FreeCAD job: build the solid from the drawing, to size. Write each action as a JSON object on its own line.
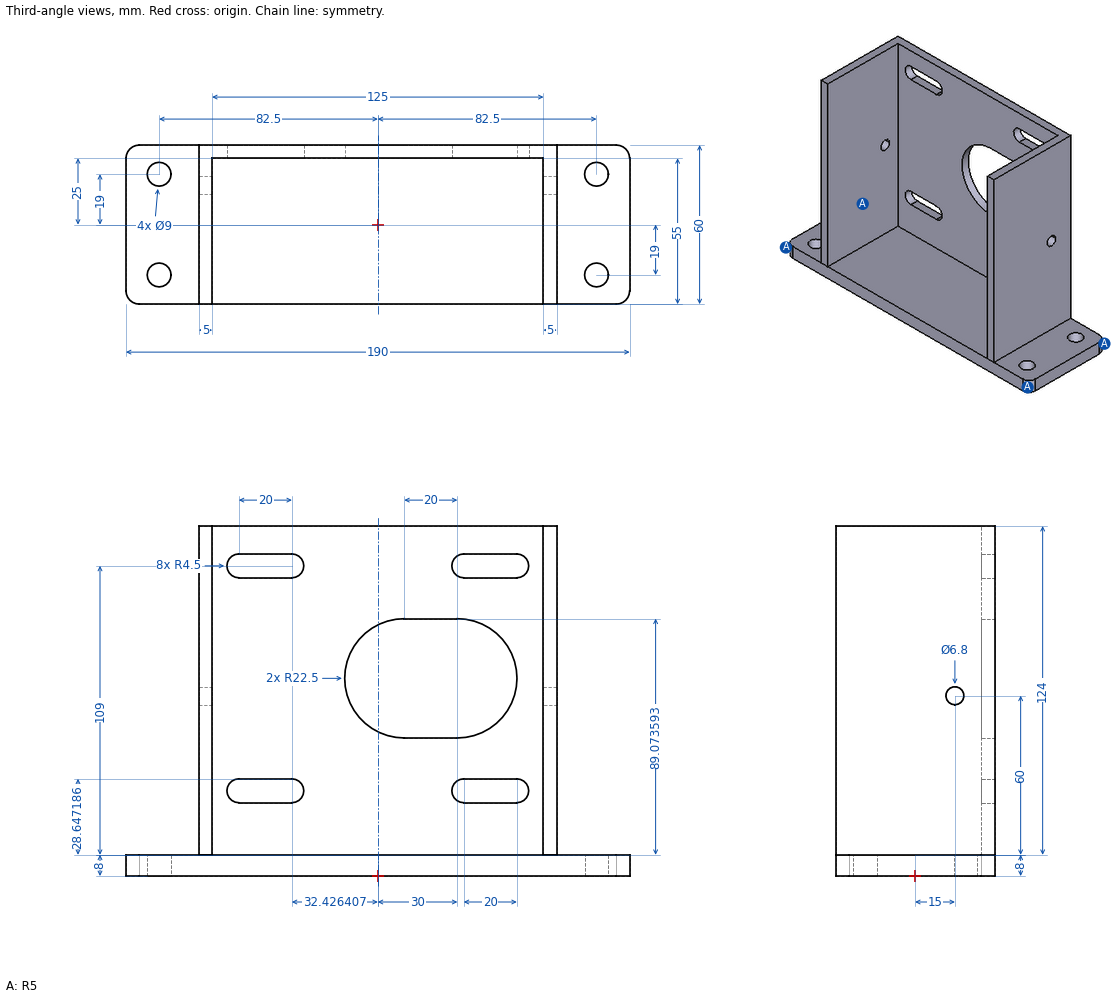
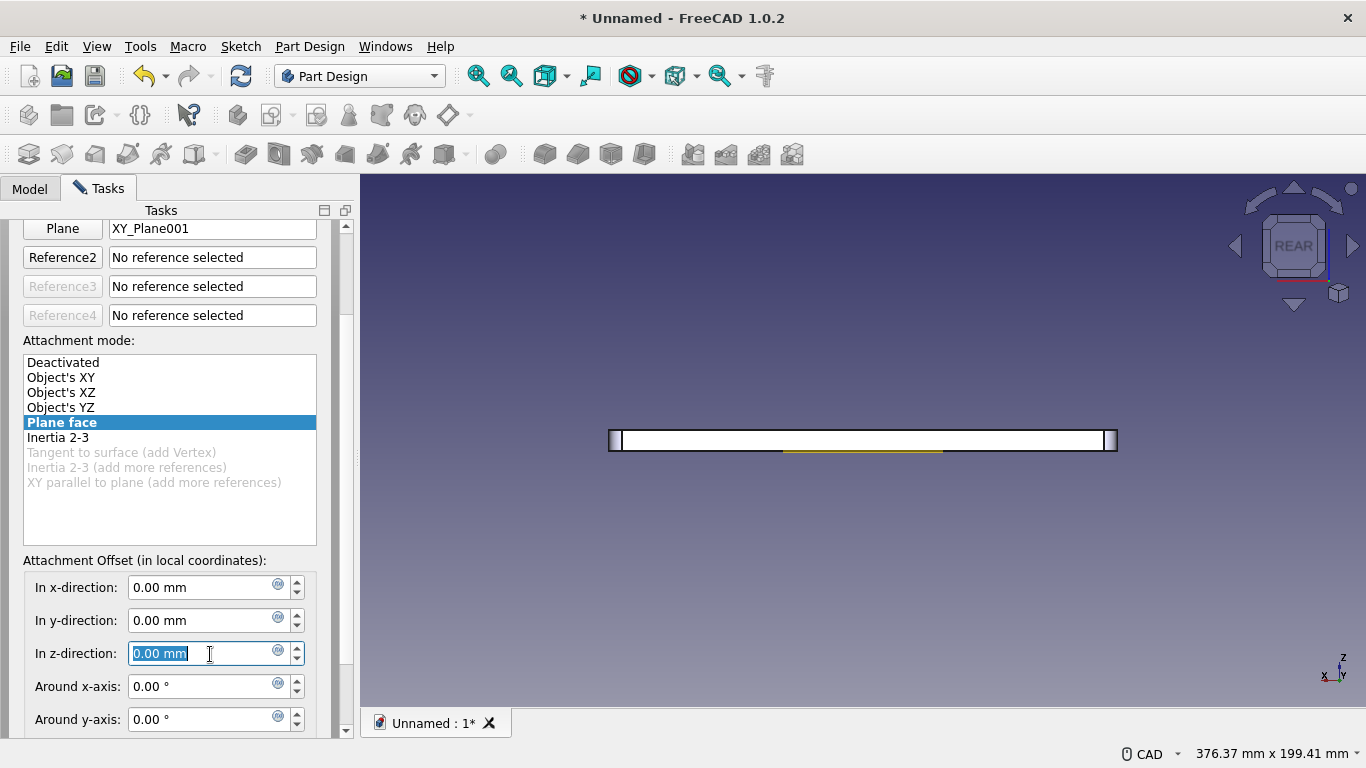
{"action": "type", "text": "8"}
{"action": "key", "text": "Tab"}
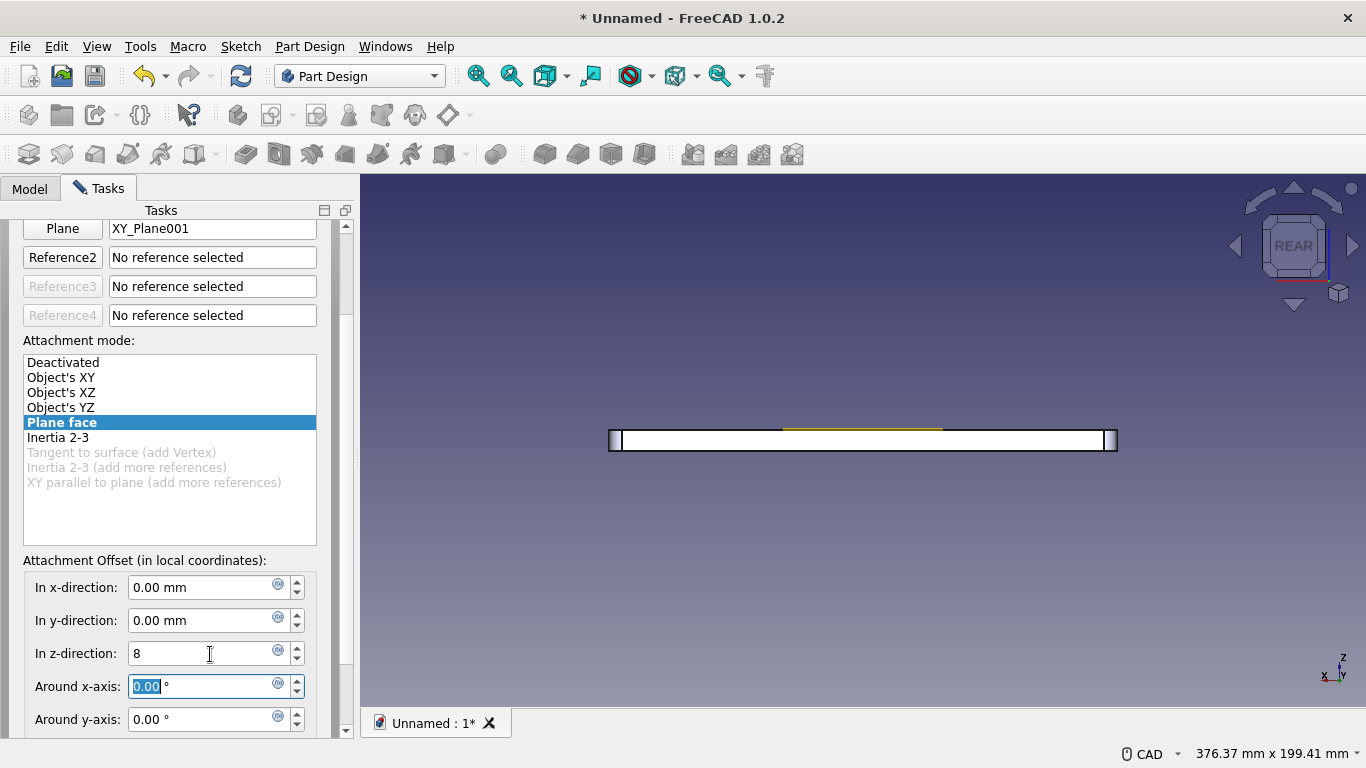
{"action": "scroll", "coordinate": [346, 479], "scroll_direction": "up", "scroll_amount": 3}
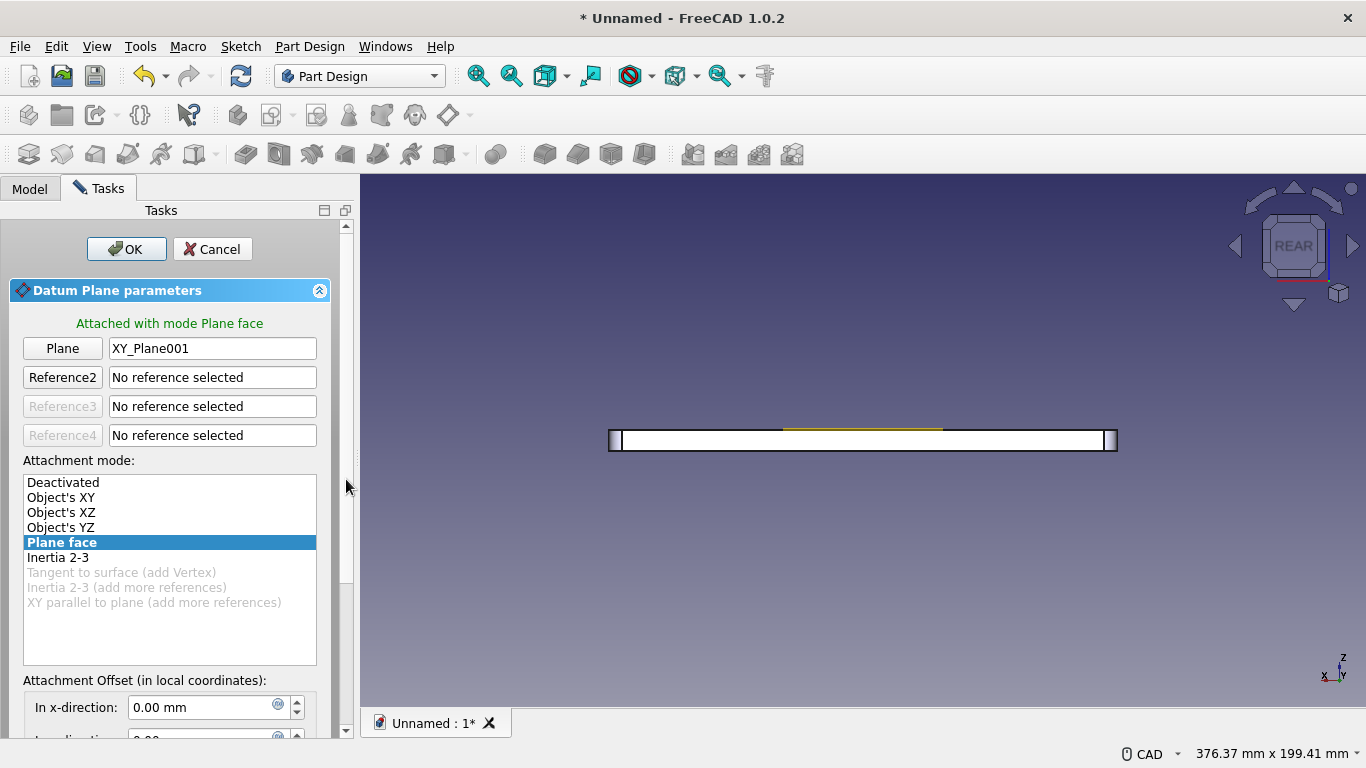
{"action": "left_click", "coordinate": [127, 249]}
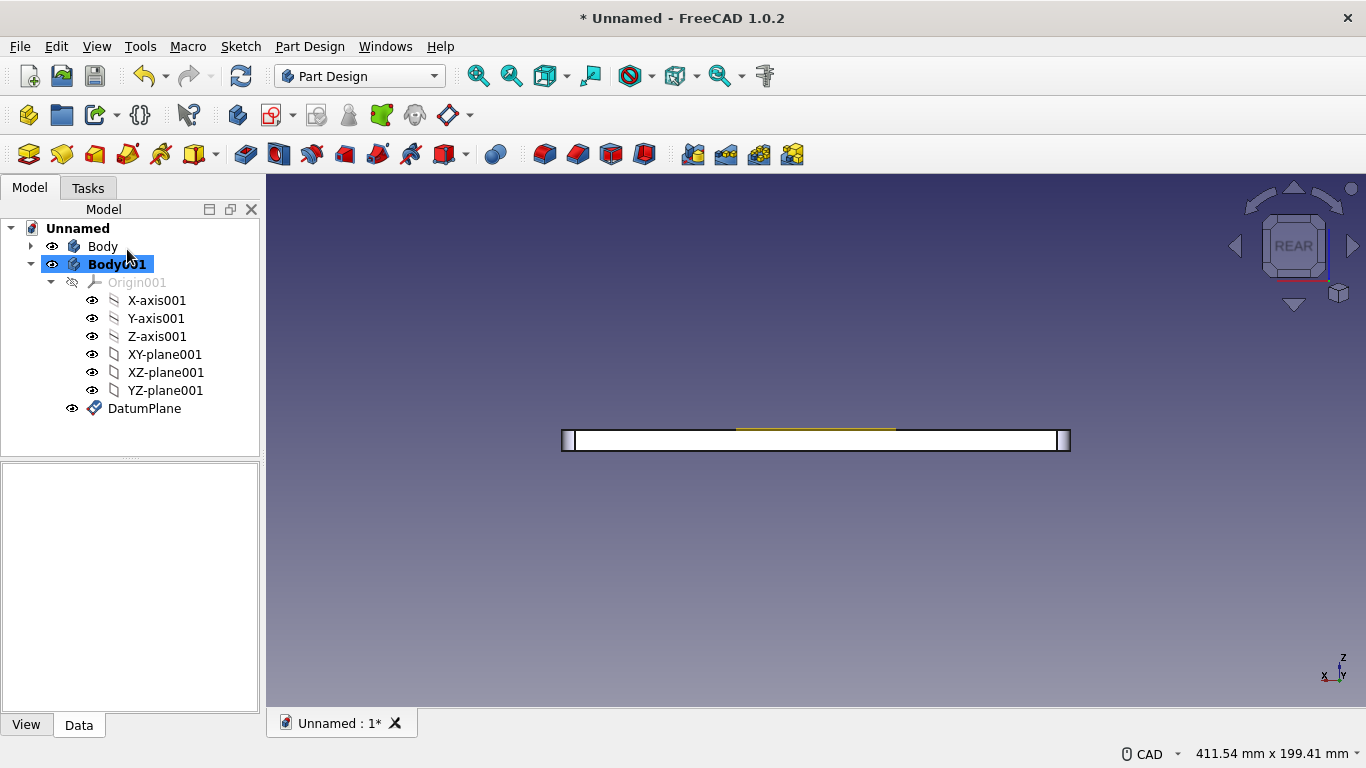
{"action": "left_click", "coordinate": [117, 408]}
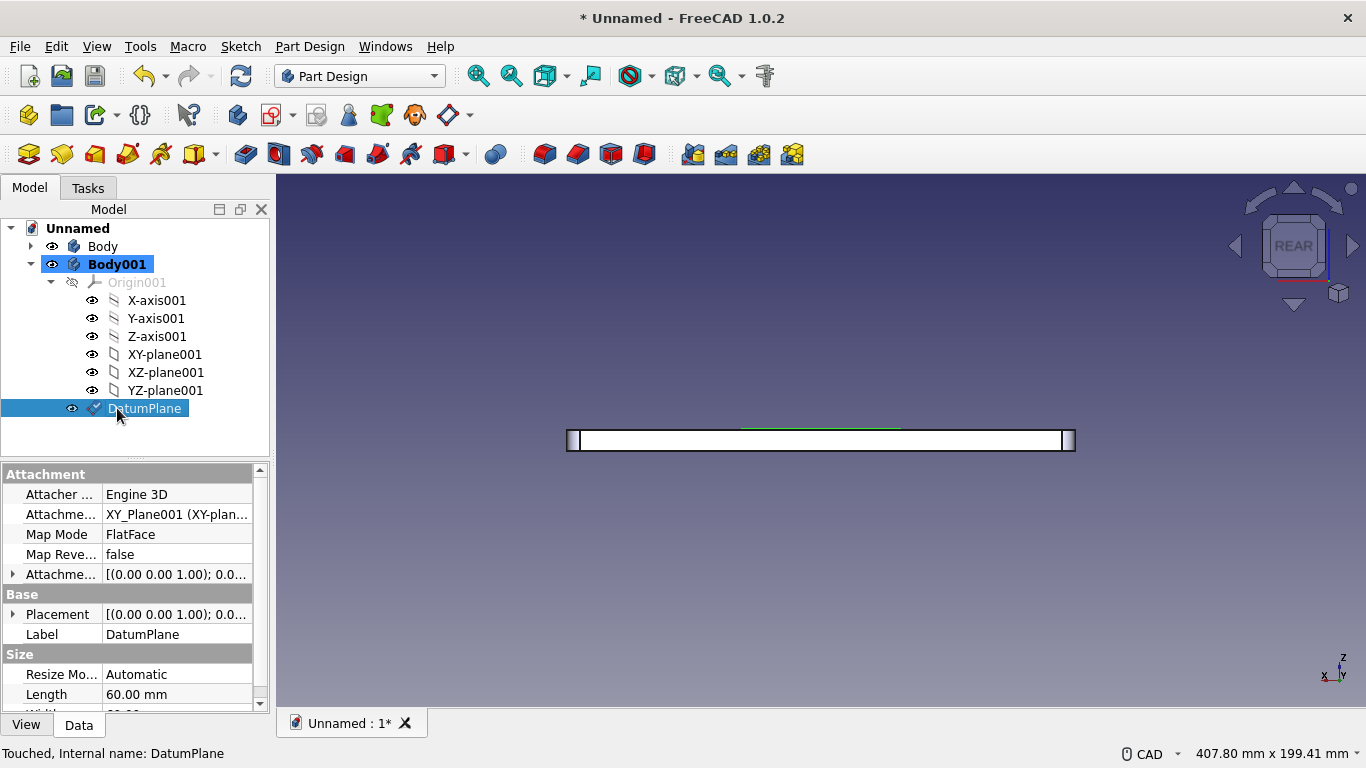
{"action": "left_click", "coordinate": [270, 116]}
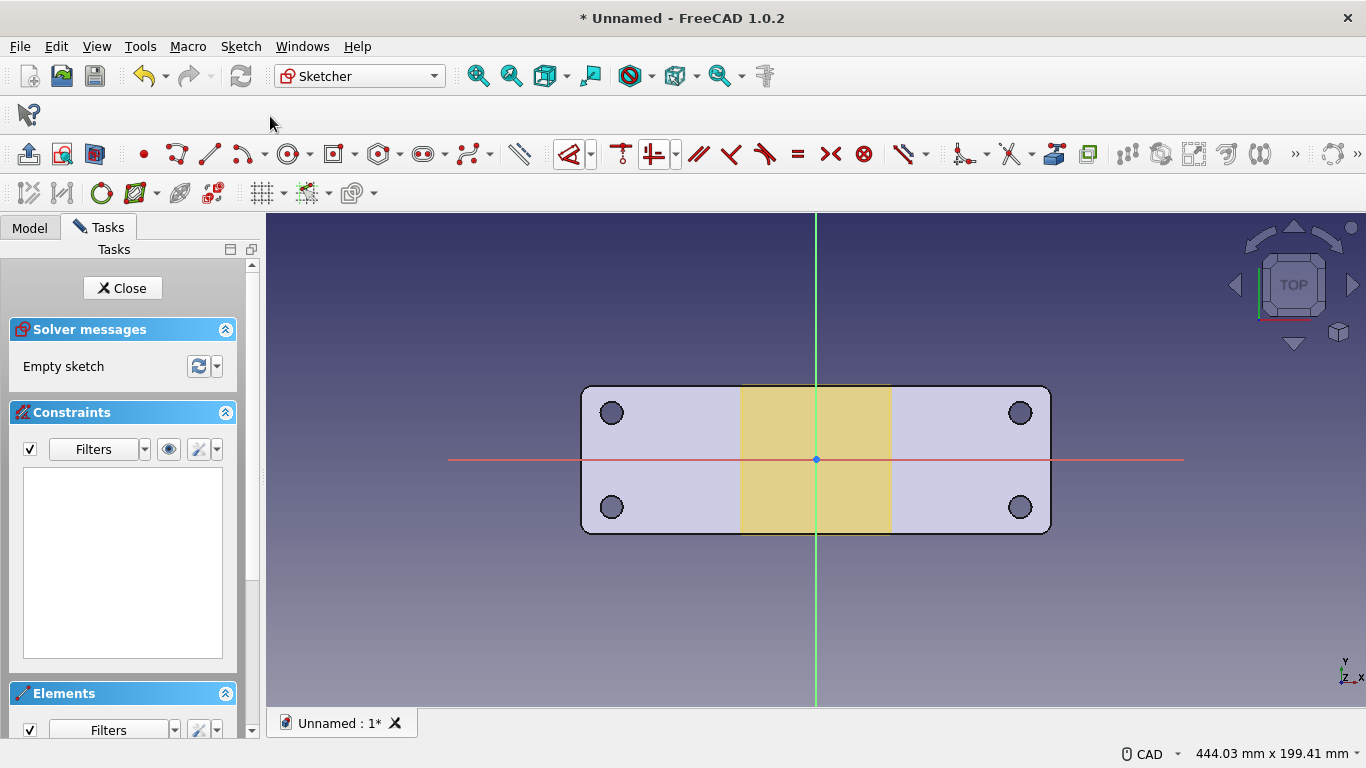
{"action": "scroll", "coordinate": [899, 460], "scroll_direction": "up", "scroll_amount": 3}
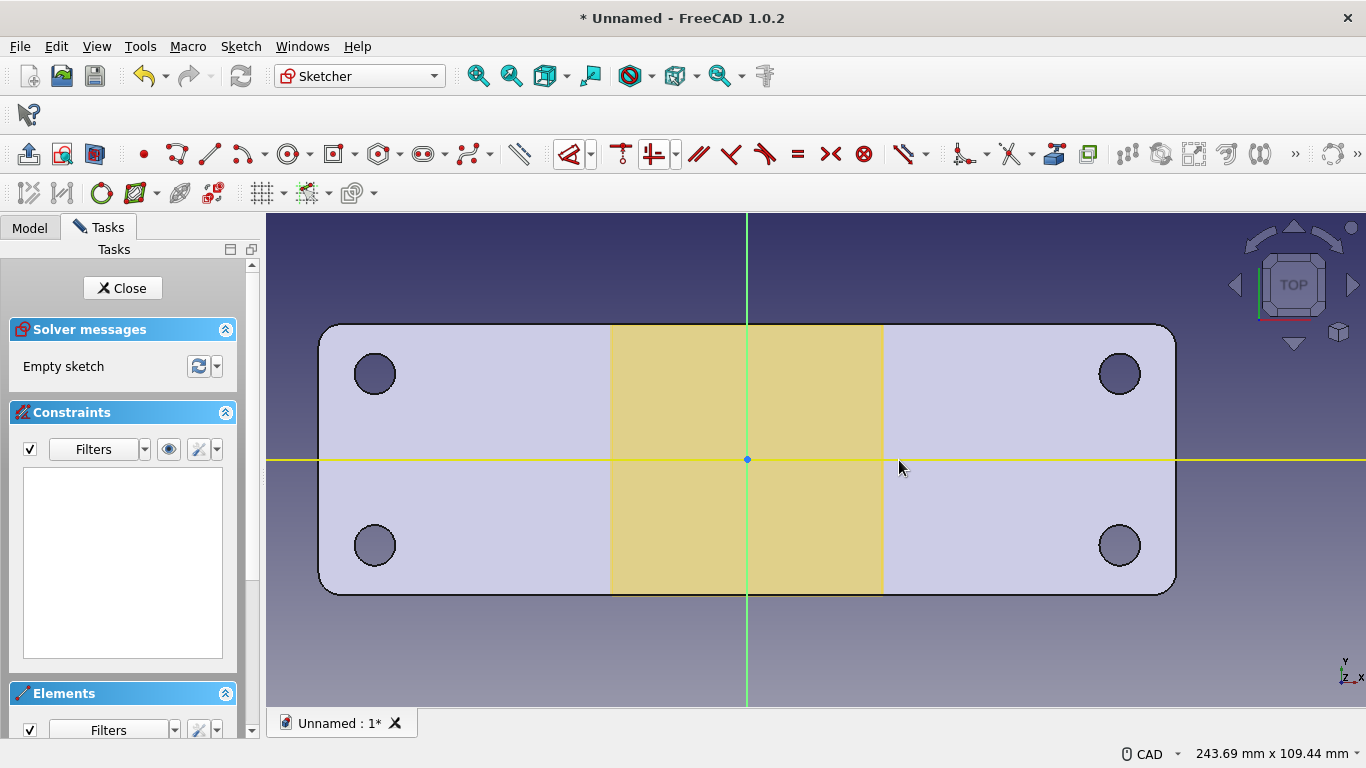
{"action": "left_click", "coordinate": [177, 154]}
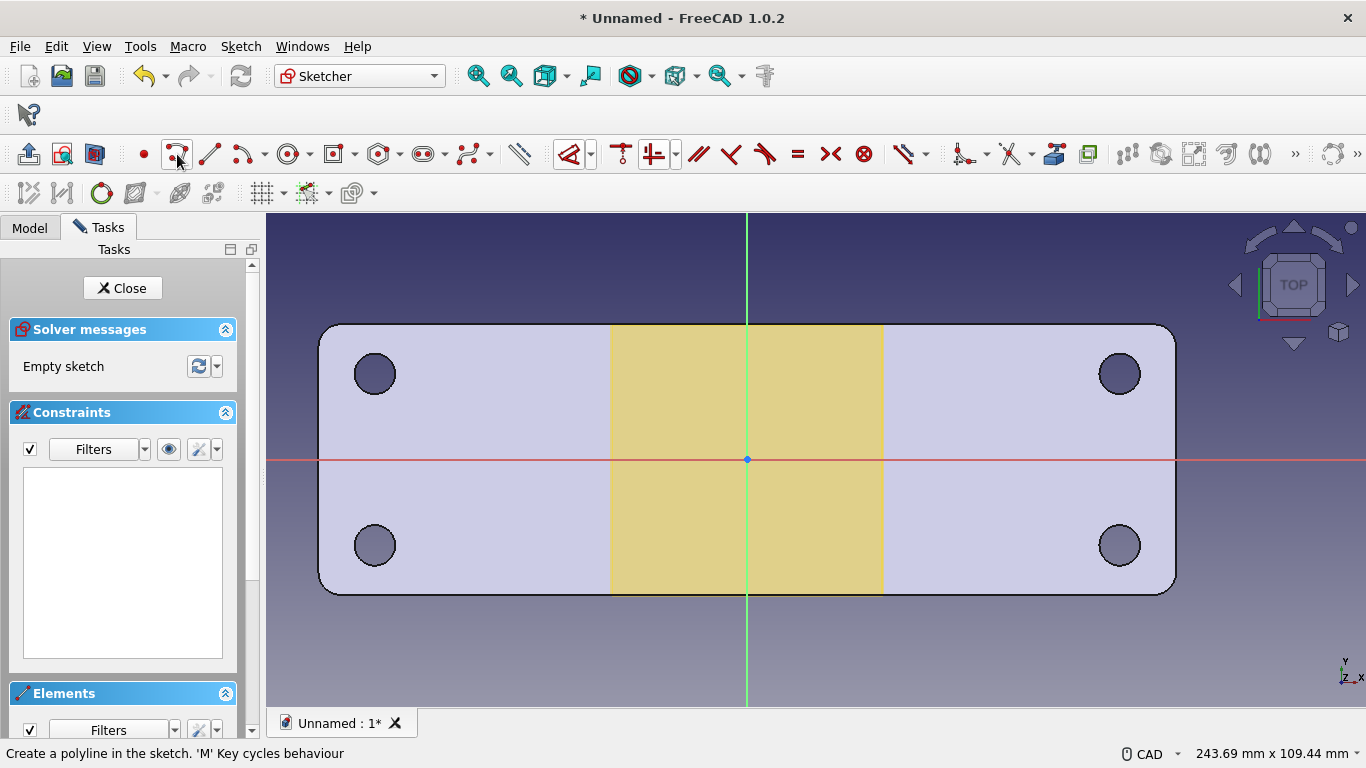
{"action": "left_click", "coordinate": [465, 347]}
{"action": "left_click", "coordinate": [1029, 347]}
{"action": "left_click", "coordinate": [1029, 595]}
{"action": "left_click", "coordinate": [1052, 595]}
{"action": "left_click", "coordinate": [1052, 324]}
{"action": "left_click", "coordinate": [443, 324]}
{"action": "left_click", "coordinate": [443, 595]}
{"action": "left_click", "coordinate": [465, 595]}
{"action": "left_click", "coordinate": [465, 348]}
{"action": "key", "text": "Escape"}
{"action": "key", "text": "Escape"}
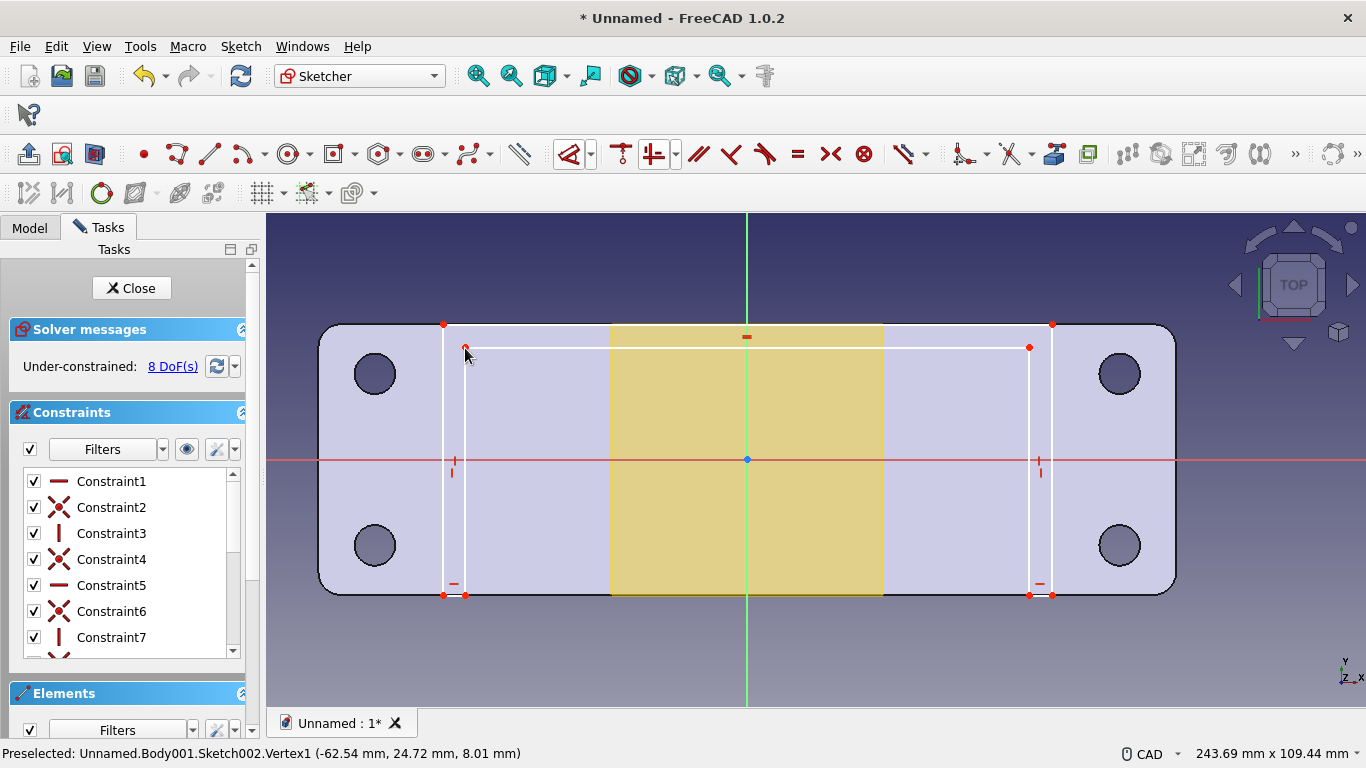
{"action": "left_click", "coordinate": [1052, 596]}